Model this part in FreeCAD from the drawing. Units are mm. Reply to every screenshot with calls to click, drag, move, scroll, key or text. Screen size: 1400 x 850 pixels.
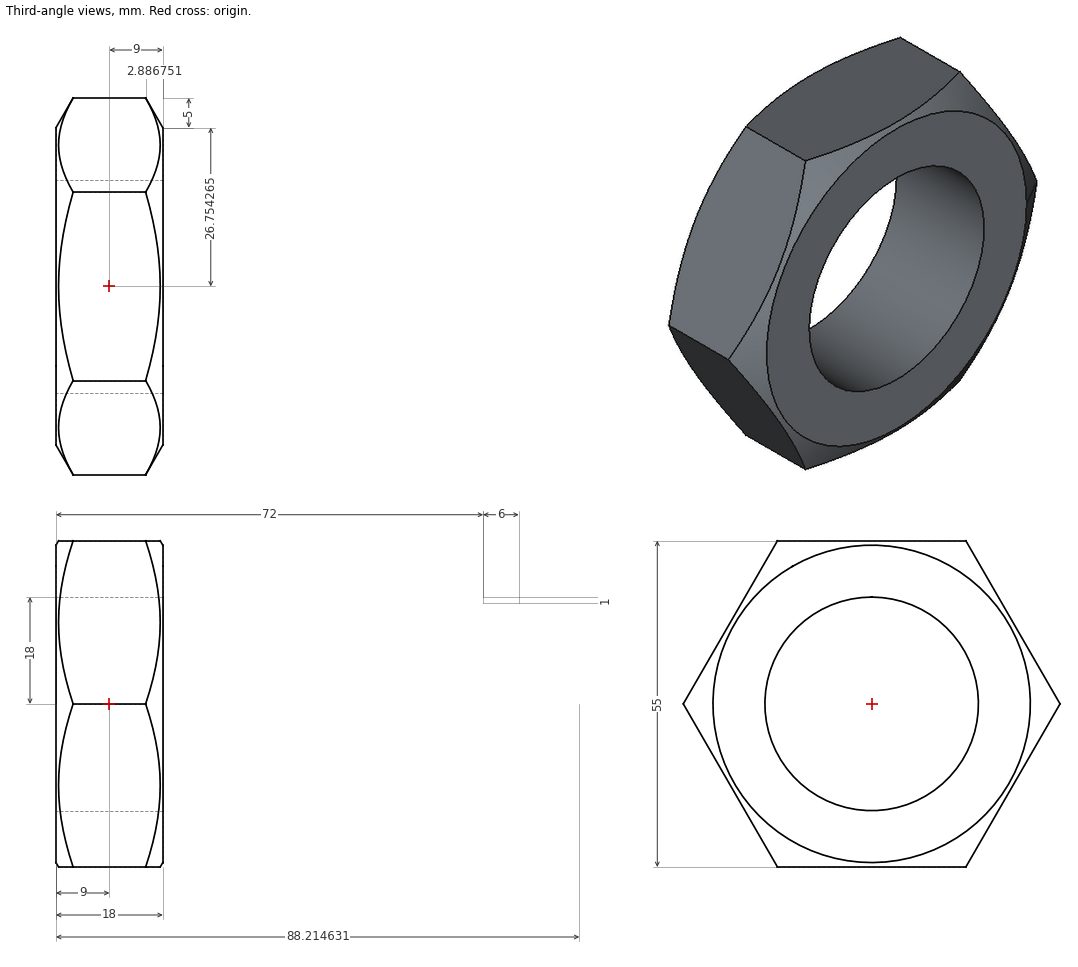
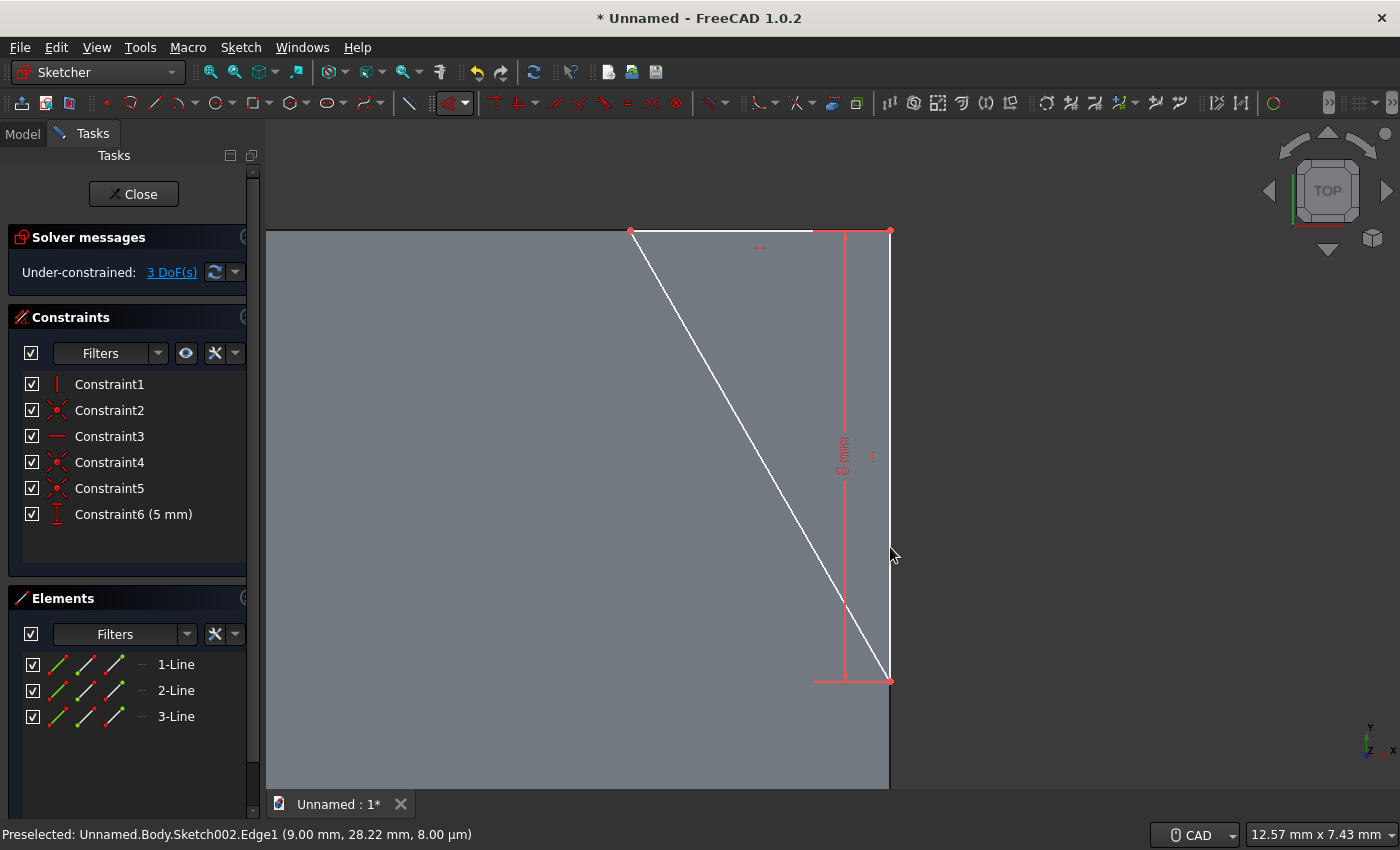
click(890, 682)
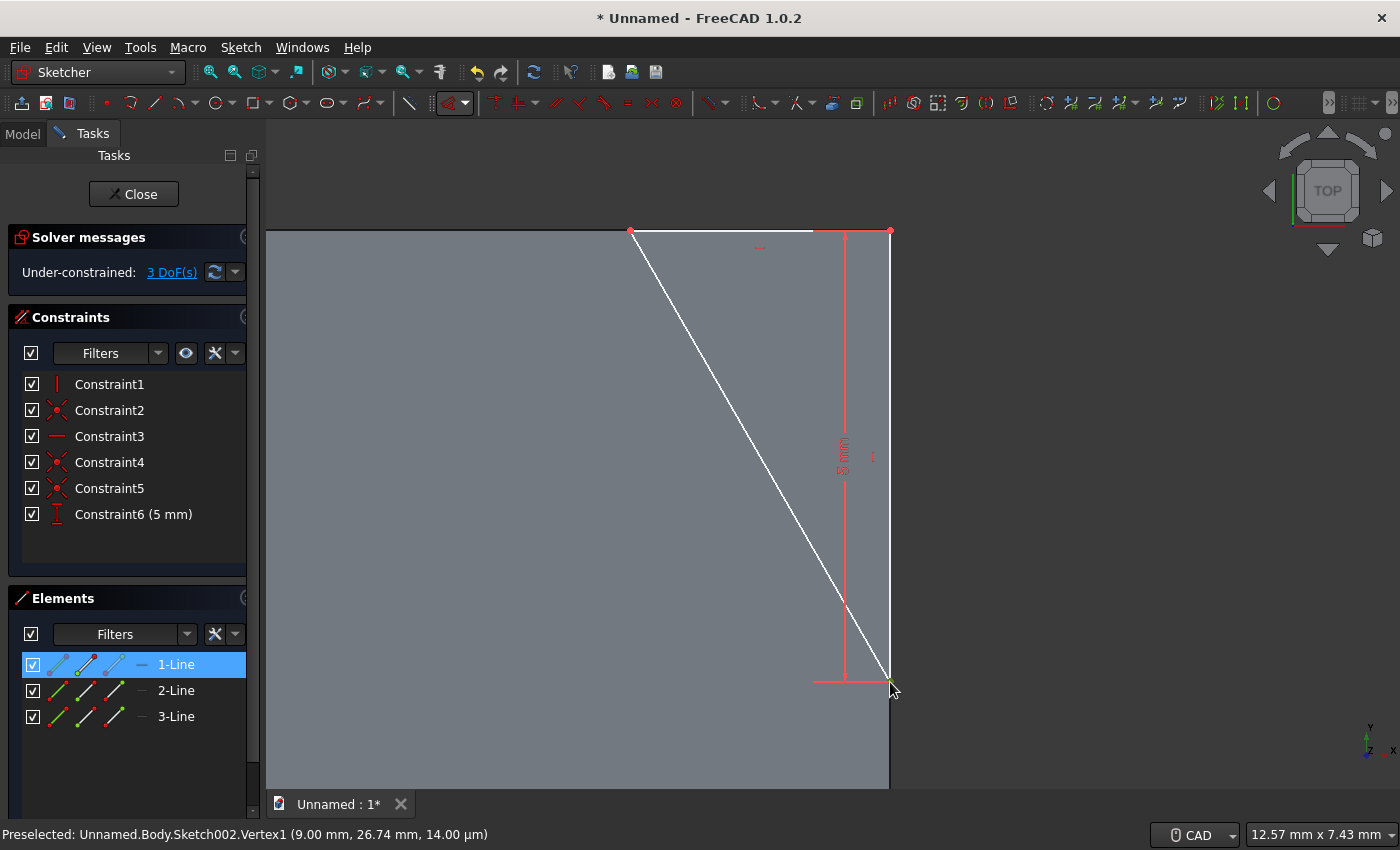
key(l)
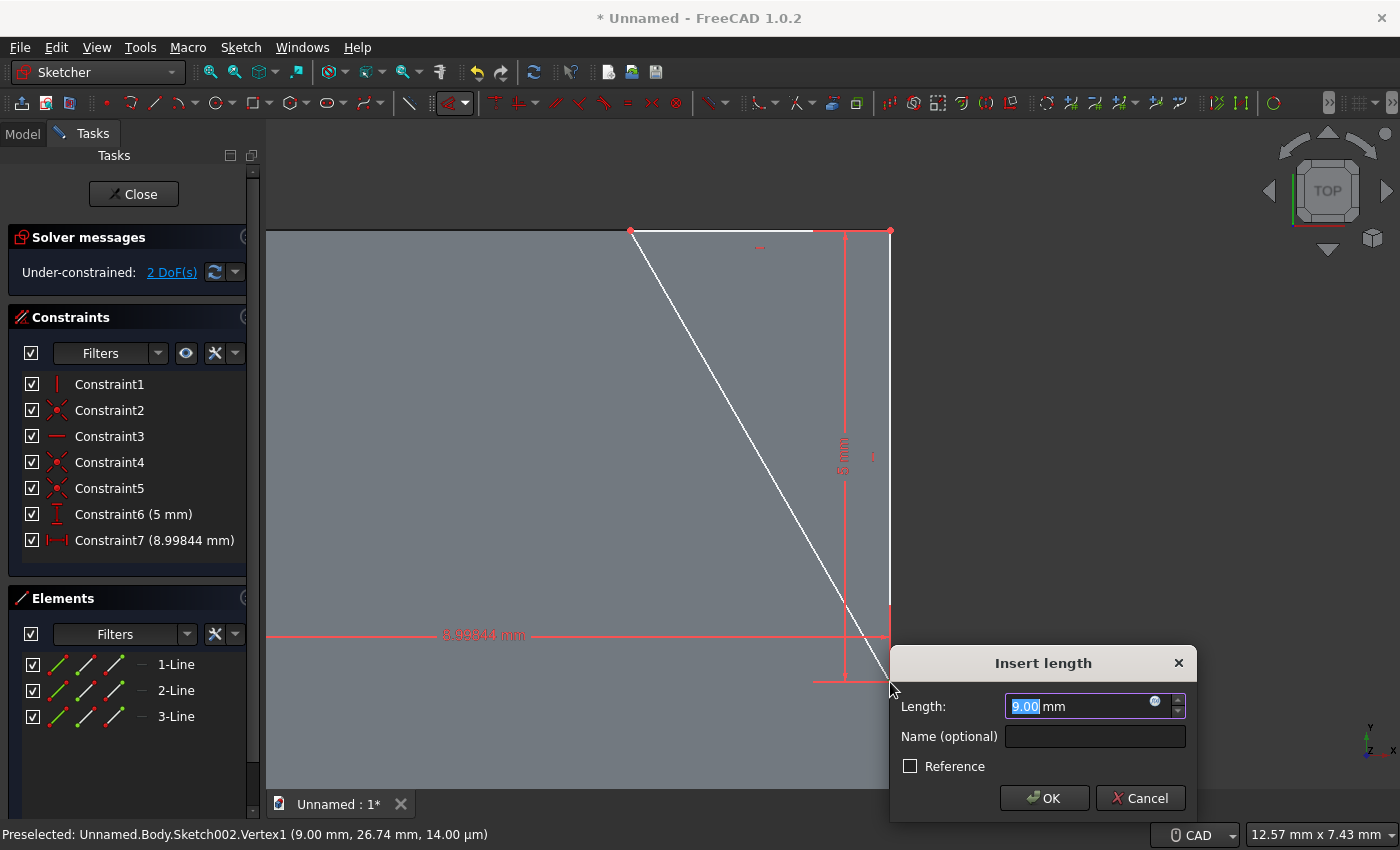
text(9)
key(Return)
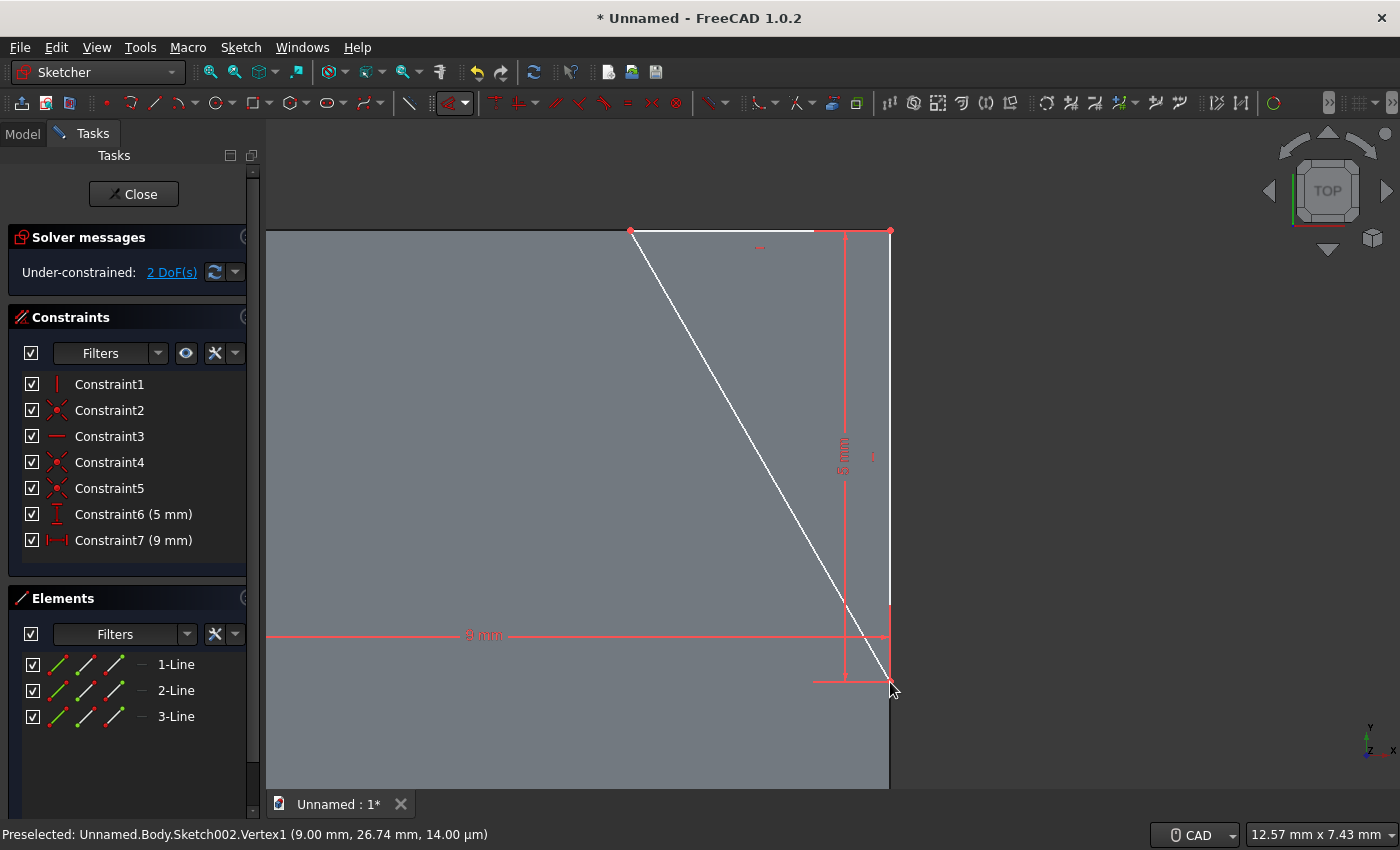
click(812, 231)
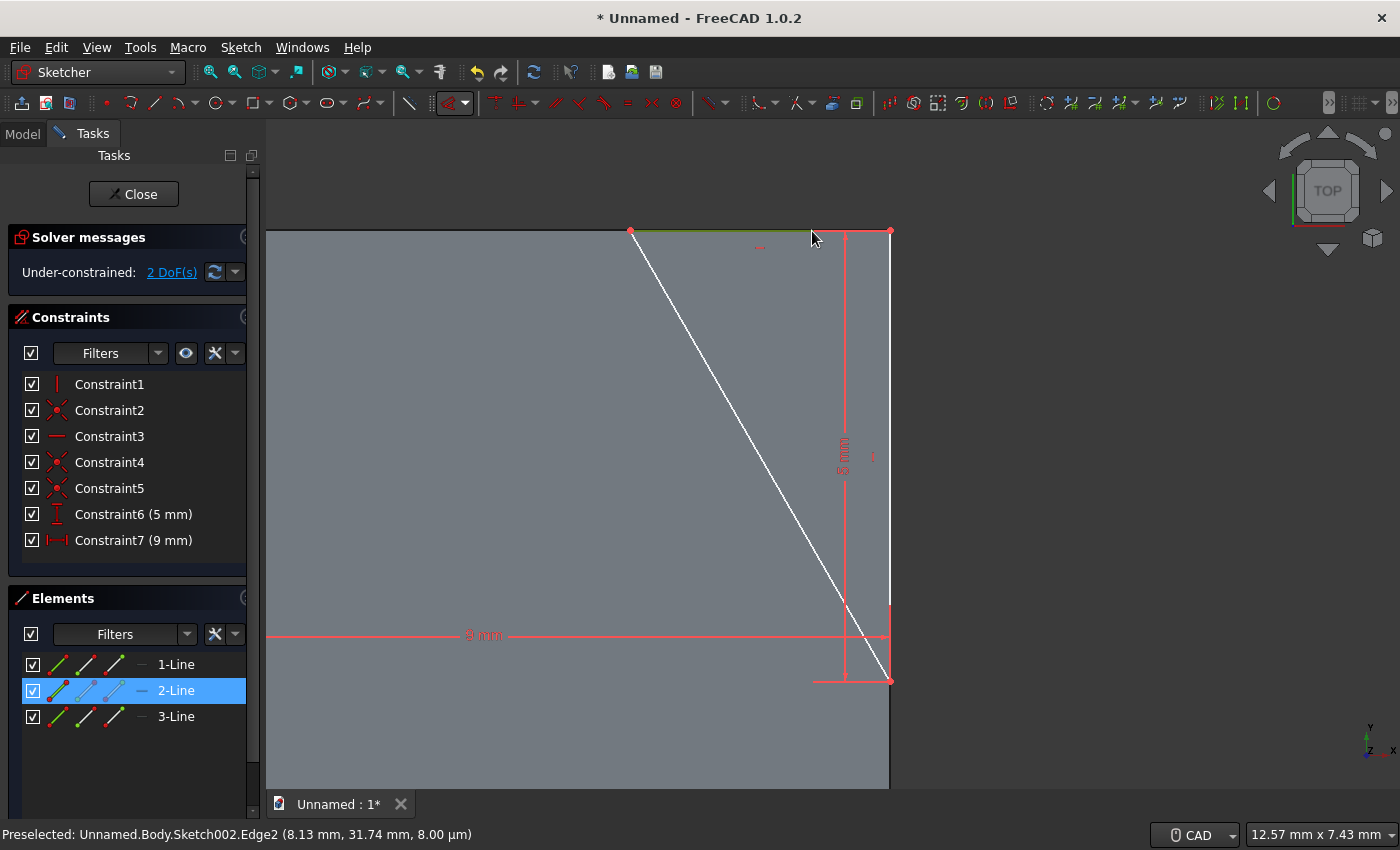
click(468, 104)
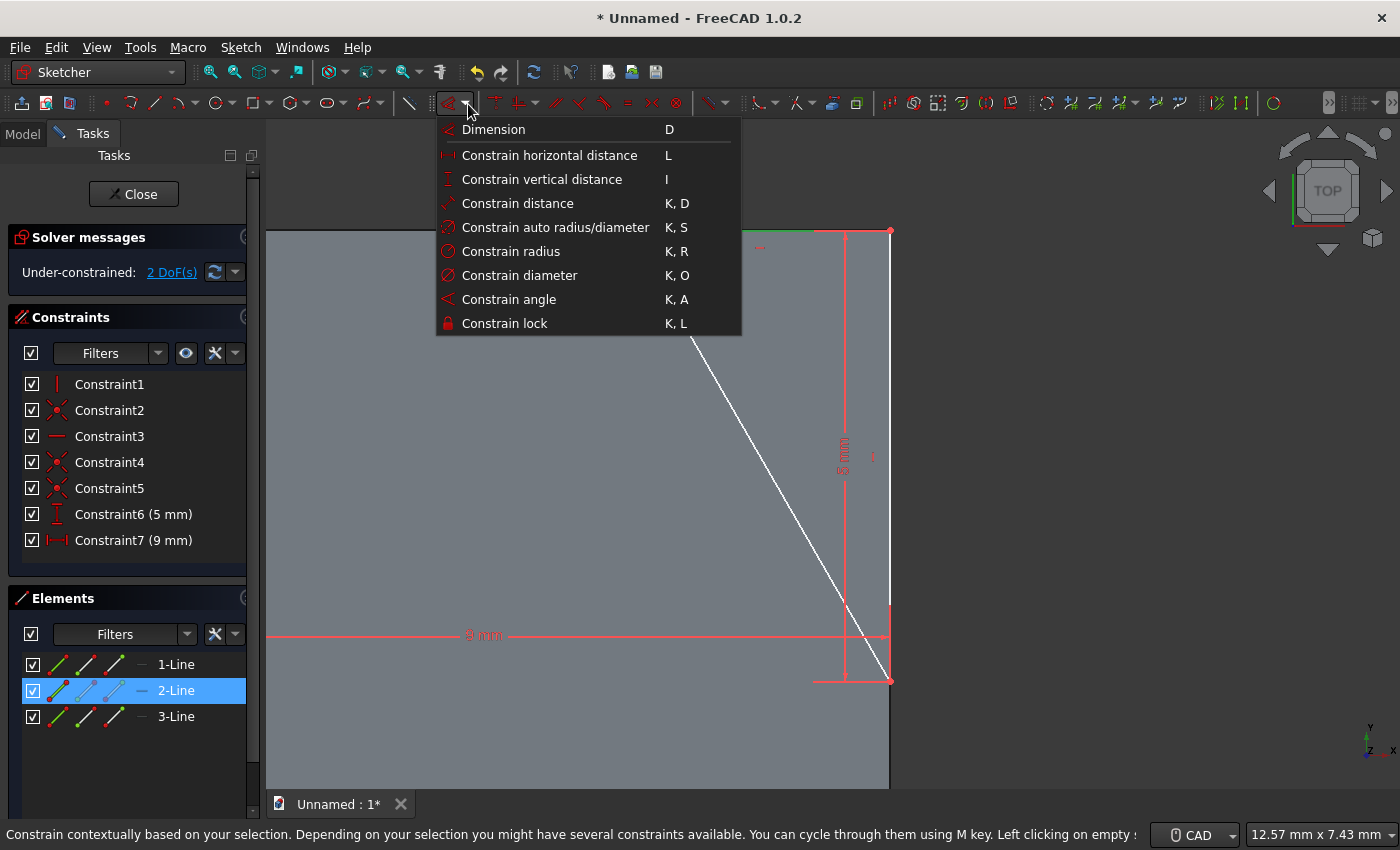
click(589, 155)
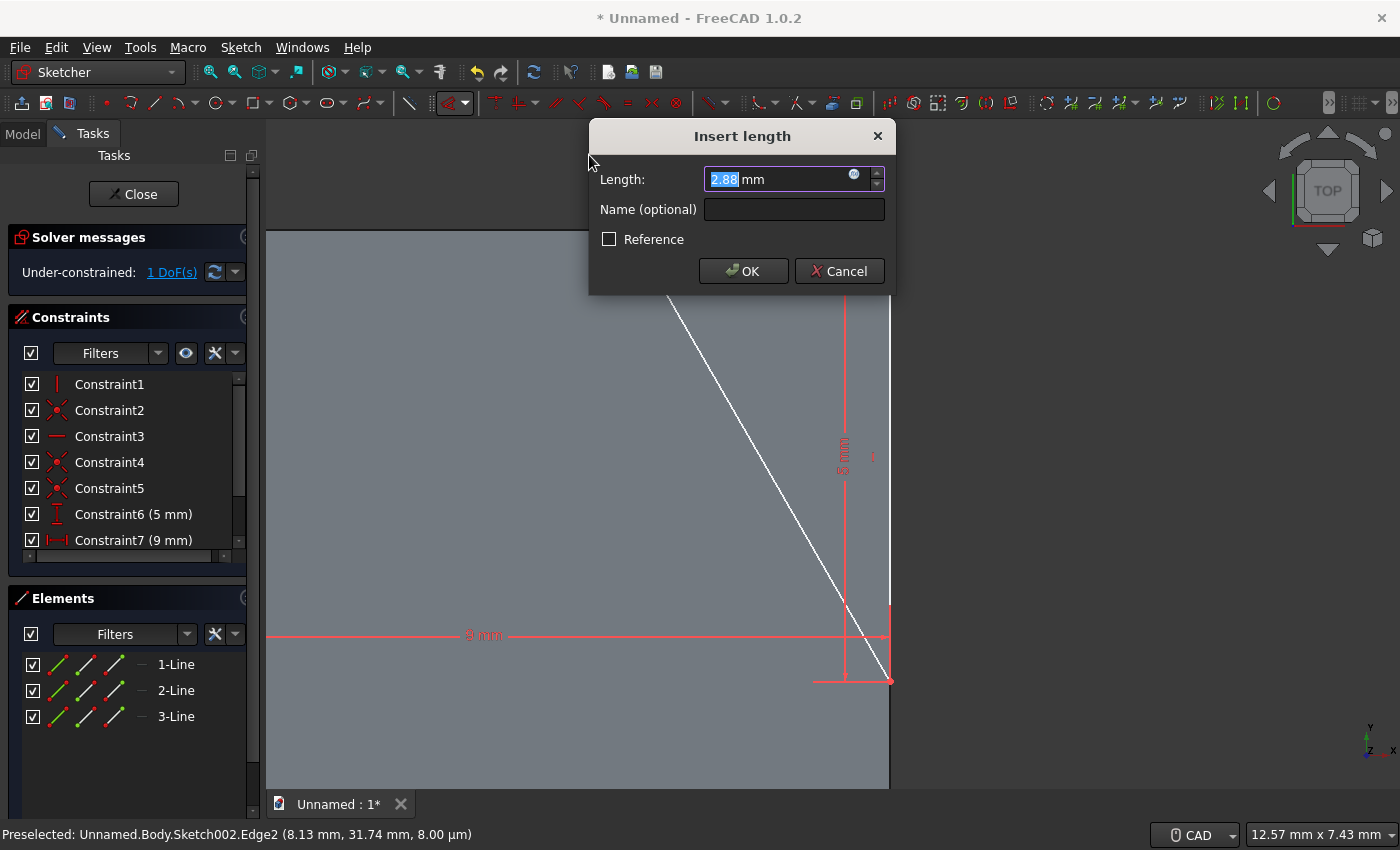
text(2.886751)
key(Return)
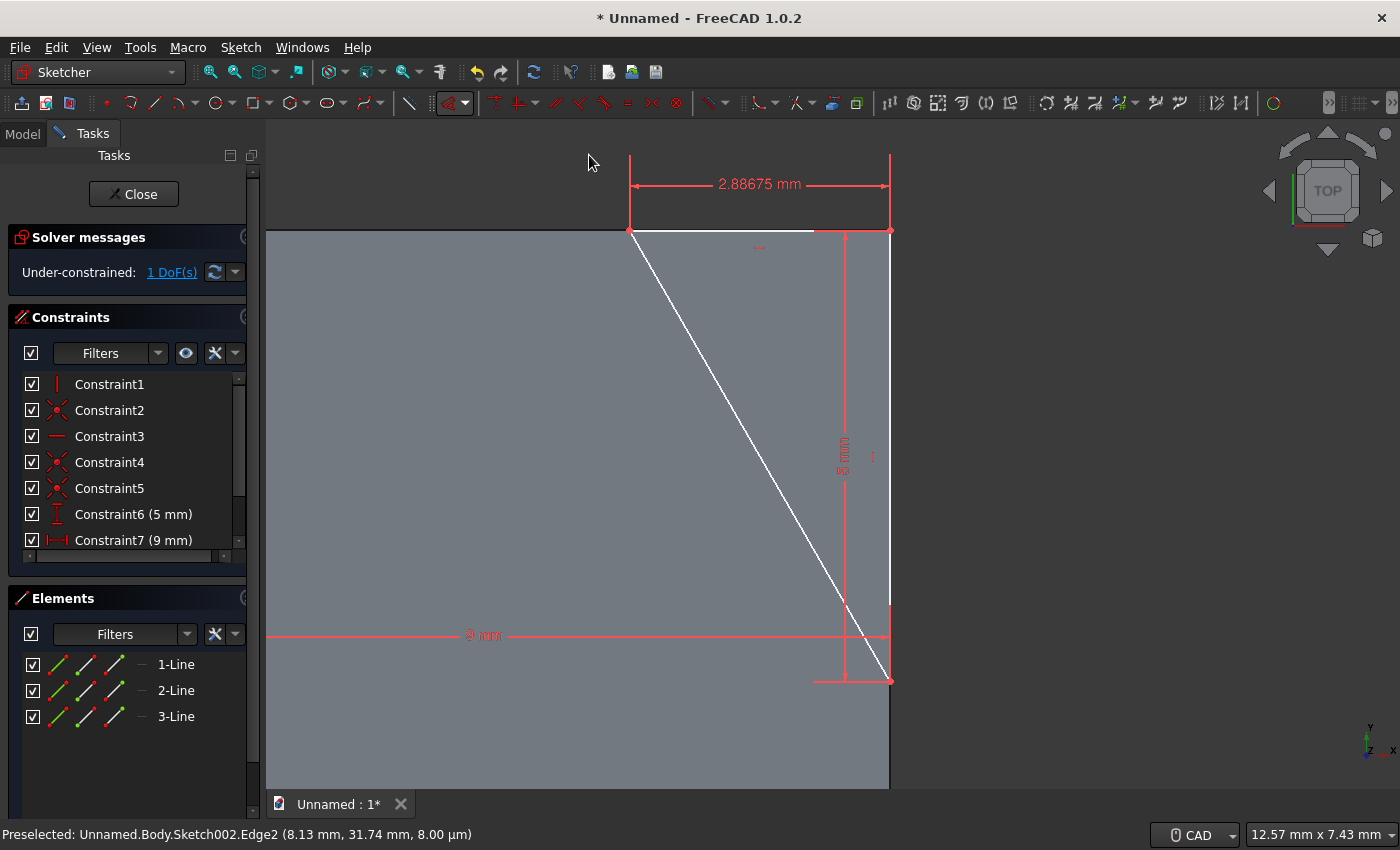
click(890, 682)